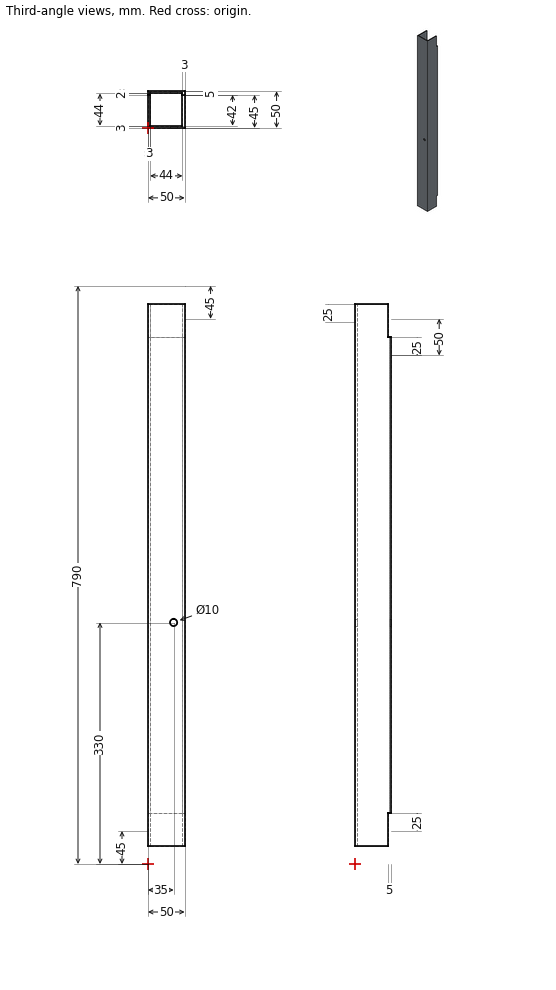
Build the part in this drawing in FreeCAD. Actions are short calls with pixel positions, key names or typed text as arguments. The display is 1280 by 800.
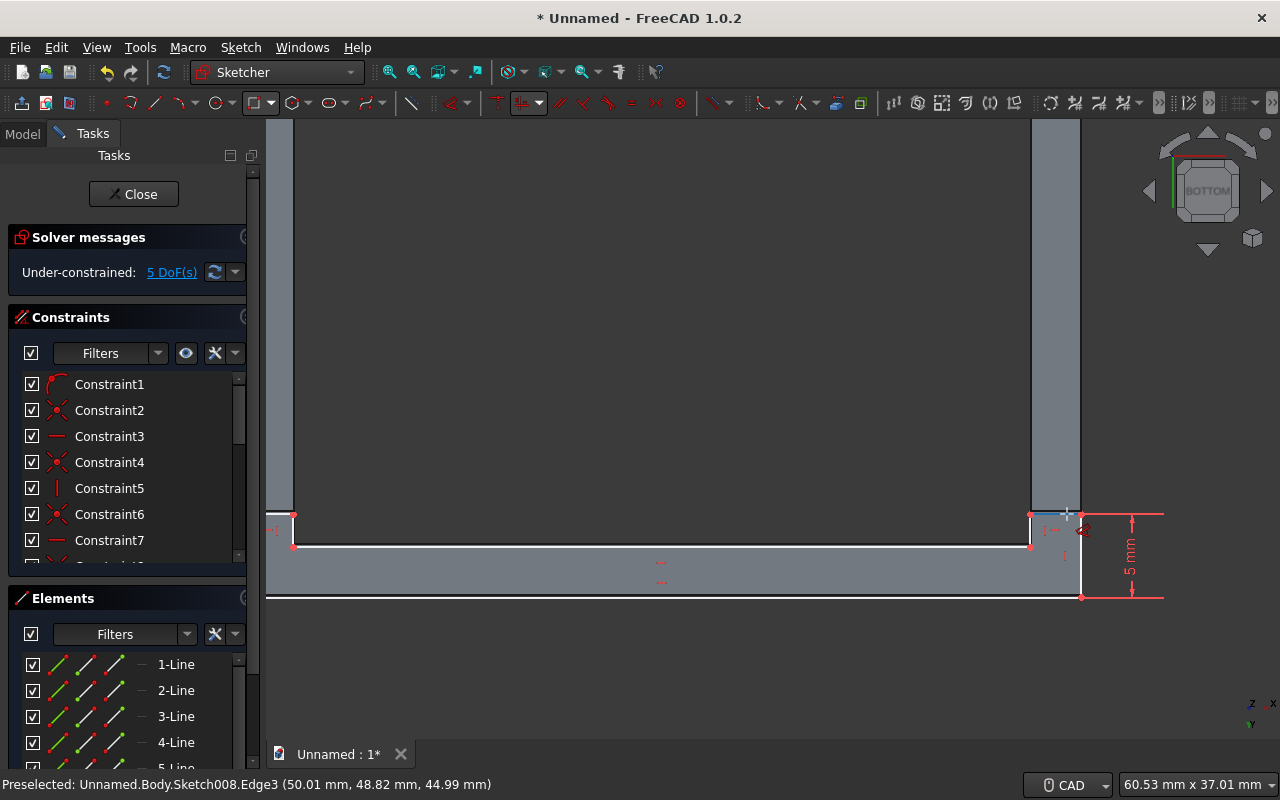
click(1066, 514)
click(1056, 548)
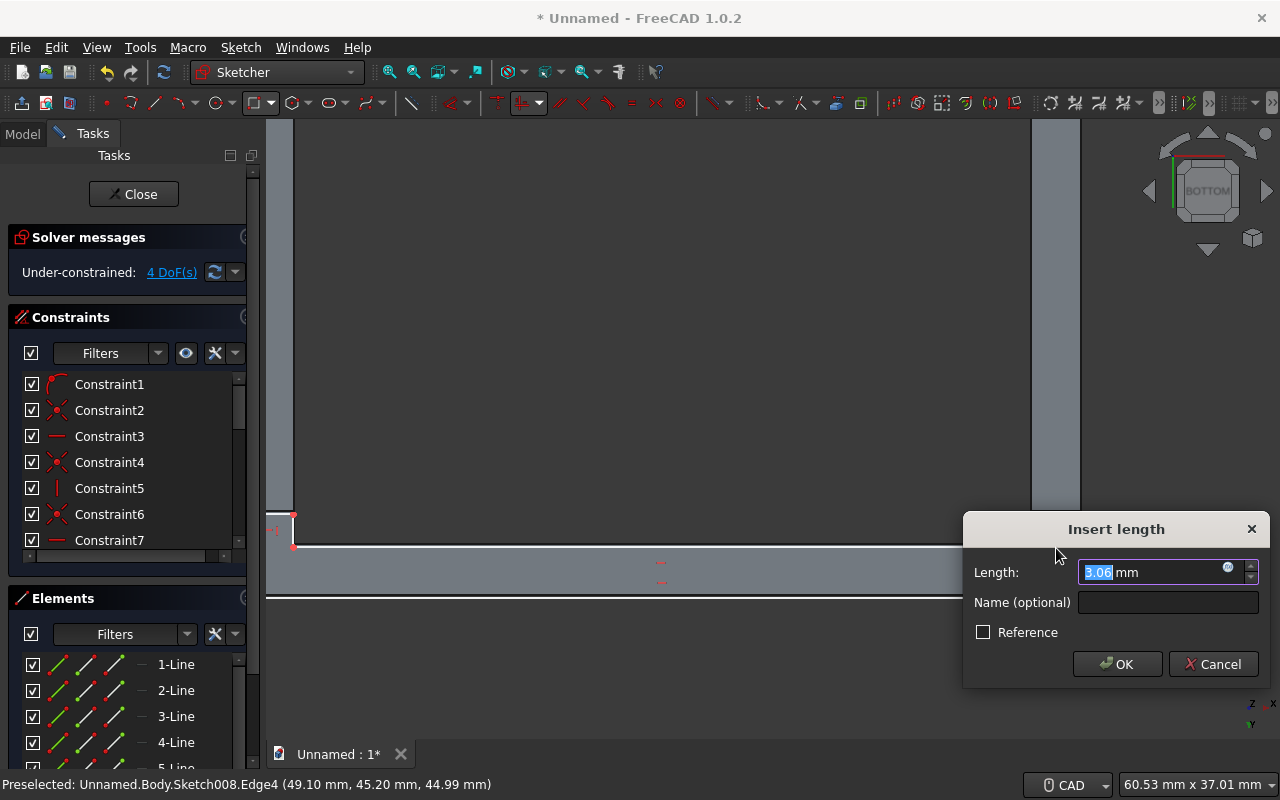
text(3)
key(Return)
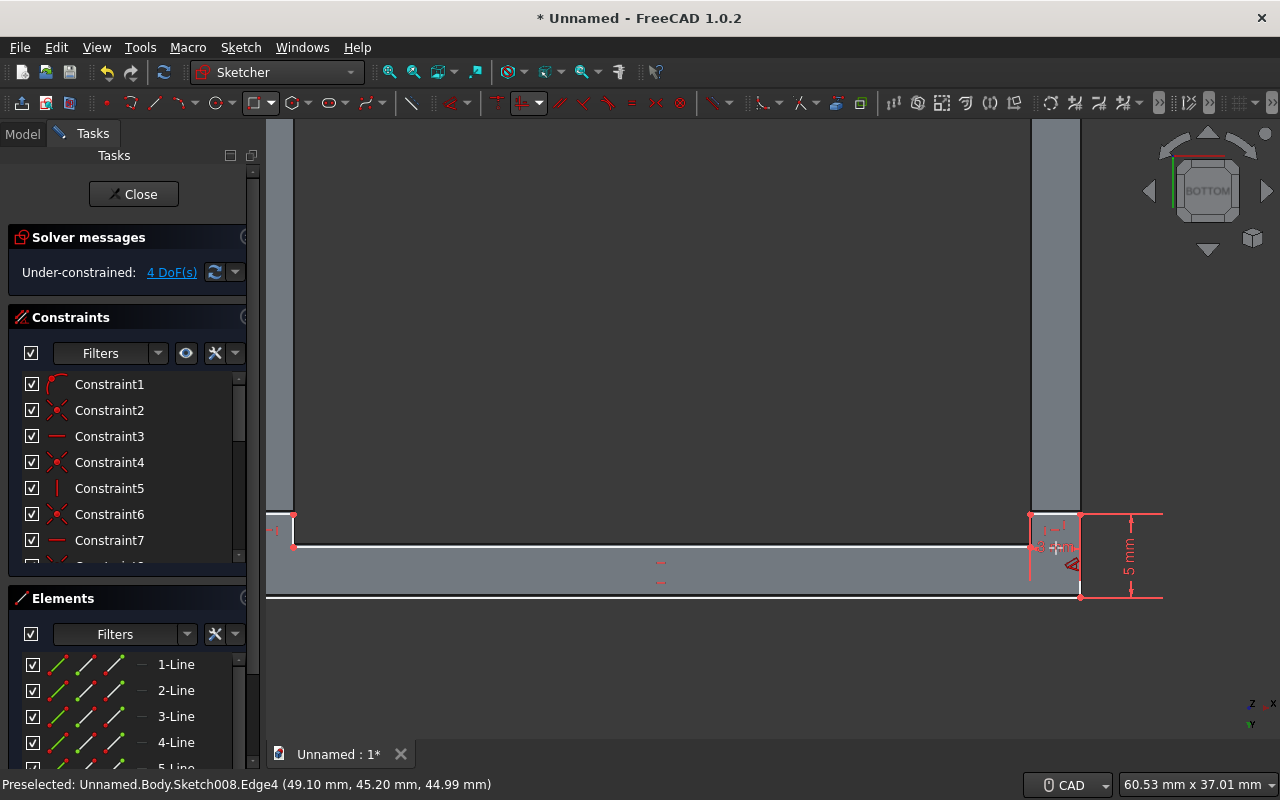
scroll(1030, 524, up, 2)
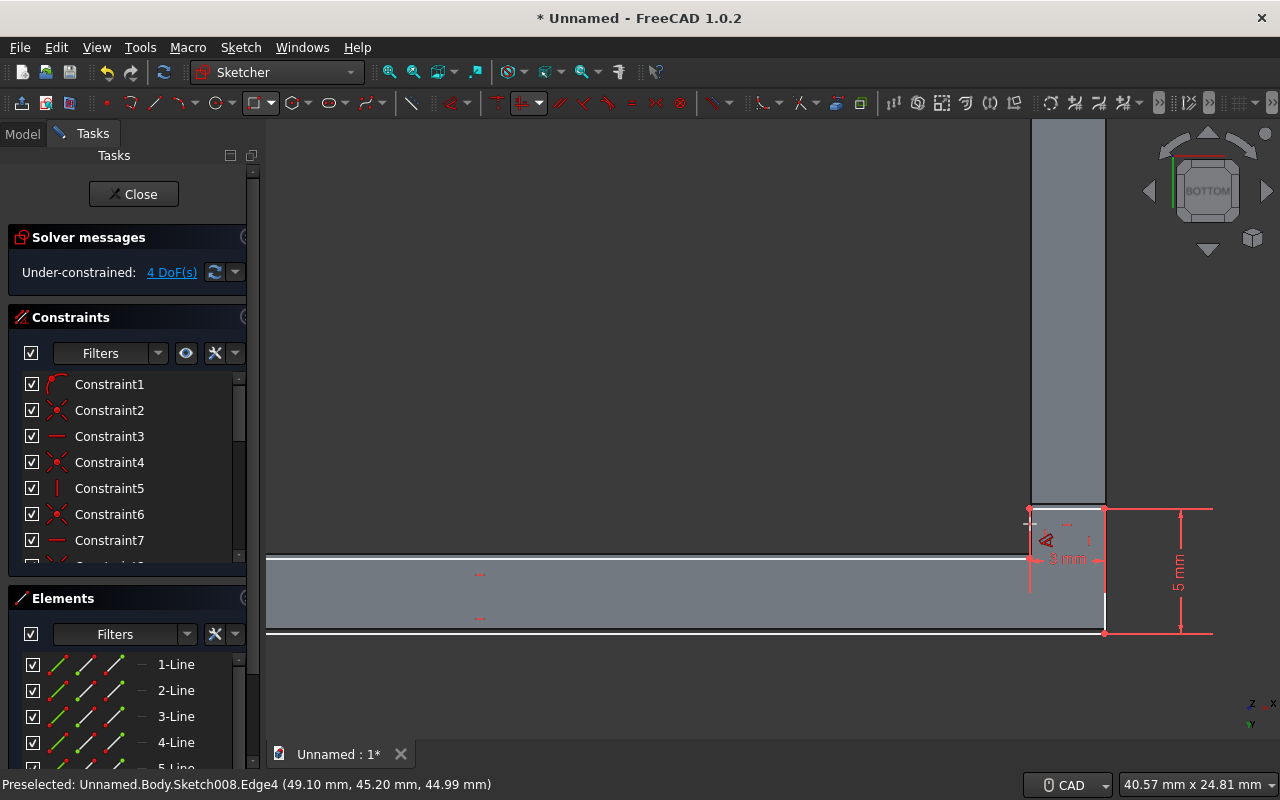
click(1030, 524)
click(1064, 534)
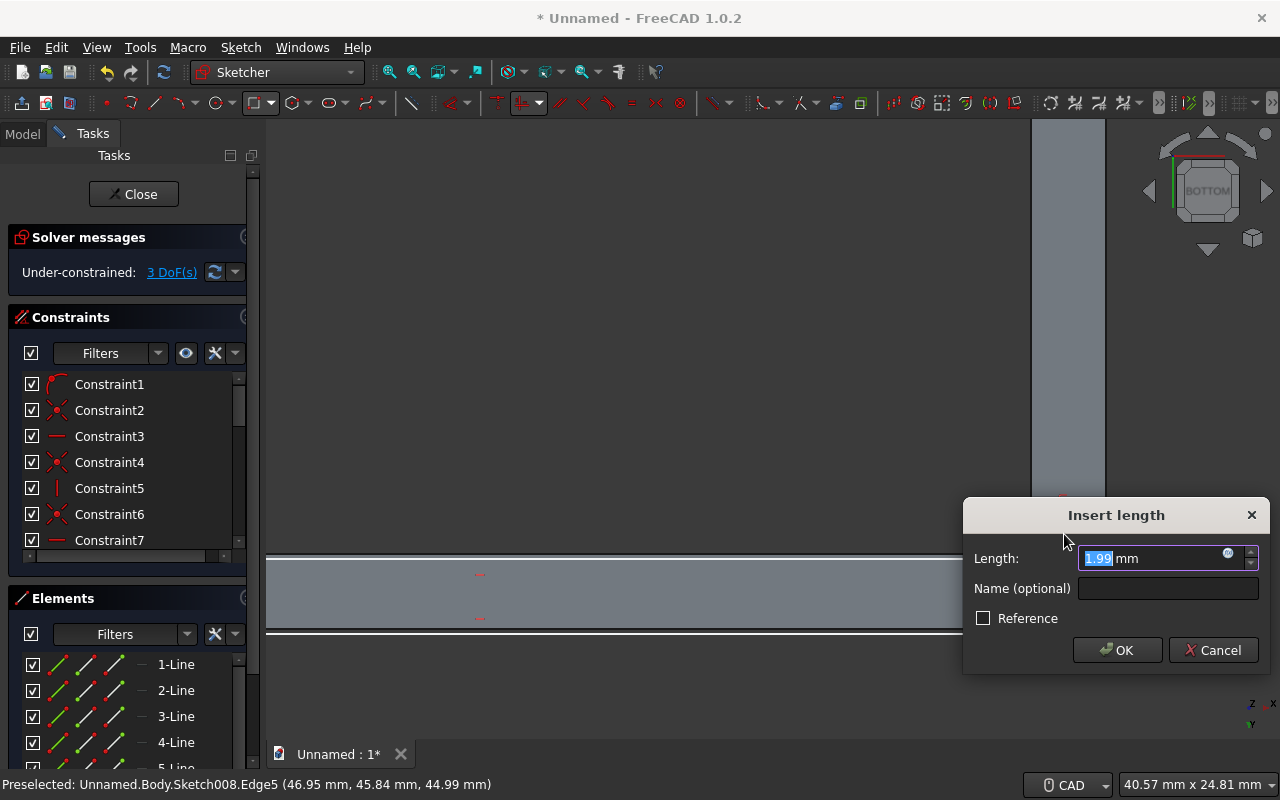
text(2)
key(Return)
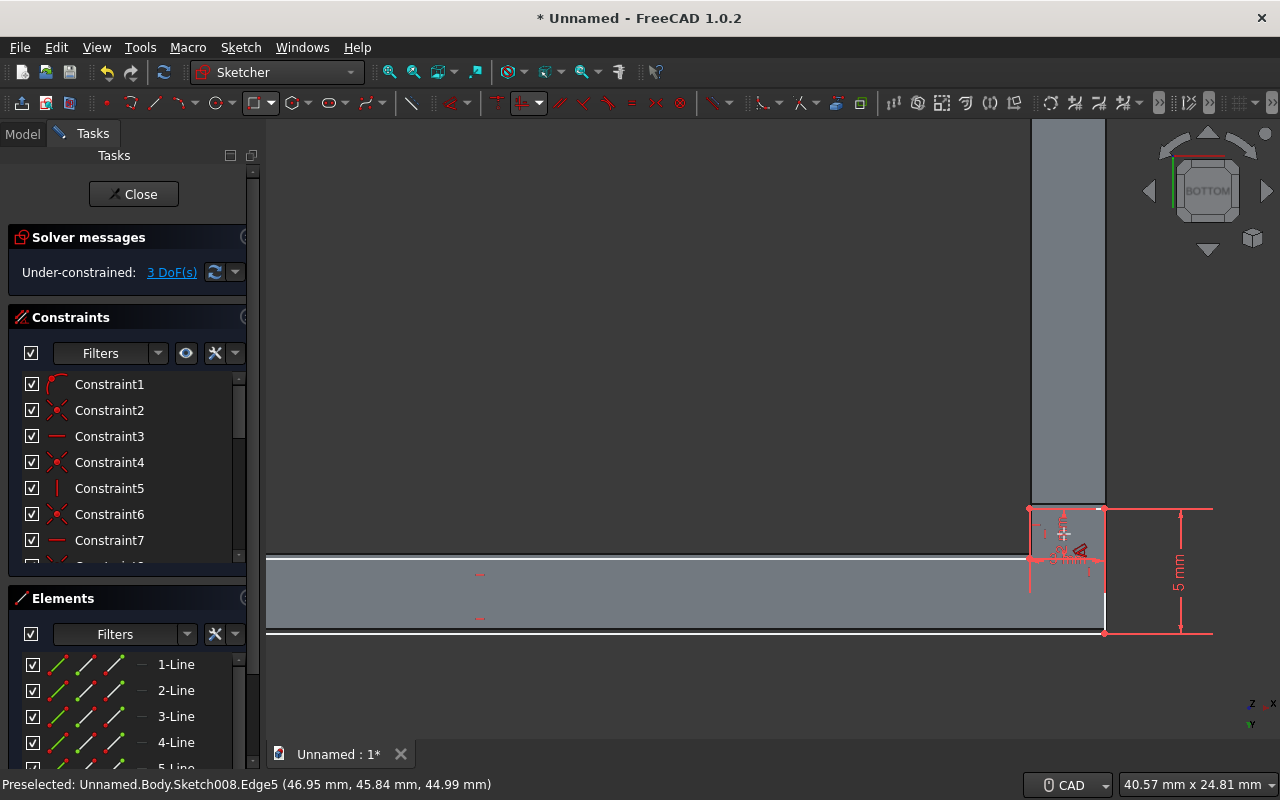
scroll(801, 612, down, 6)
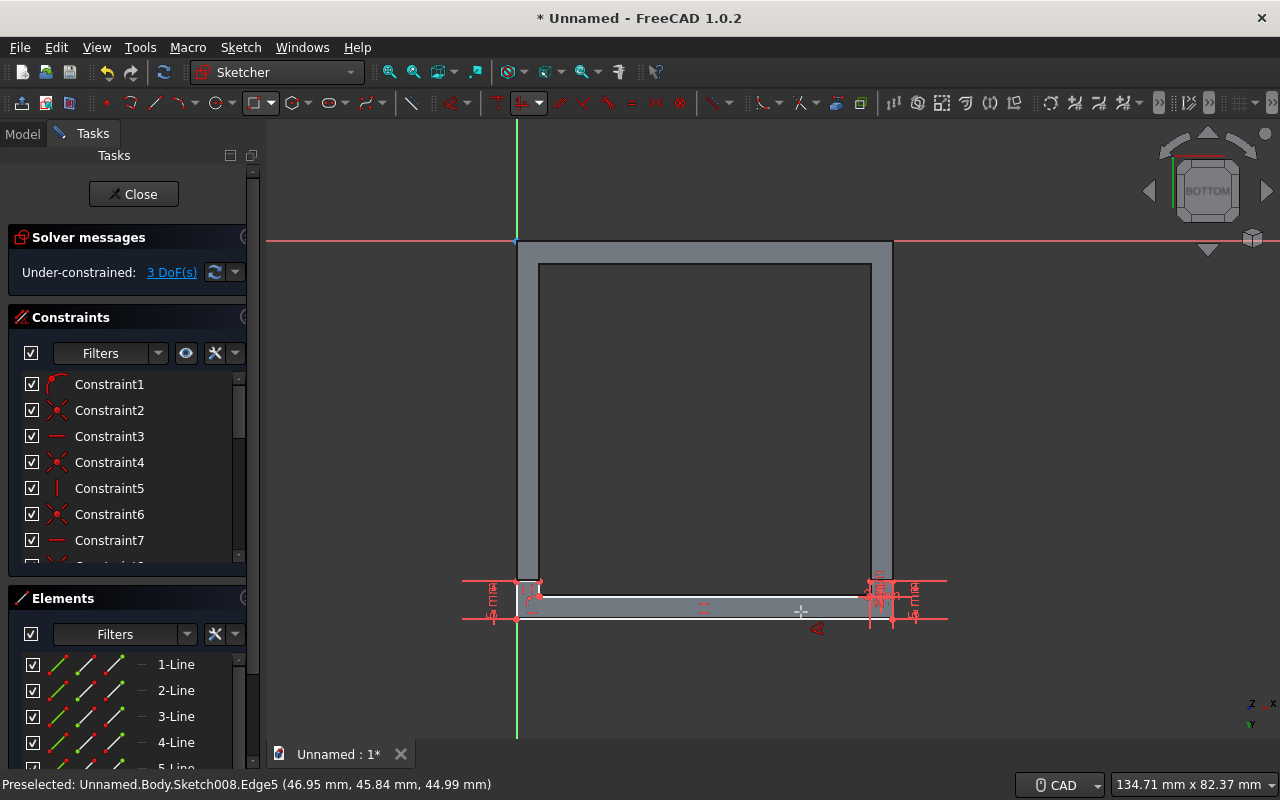
scroll(533, 581, up, 4)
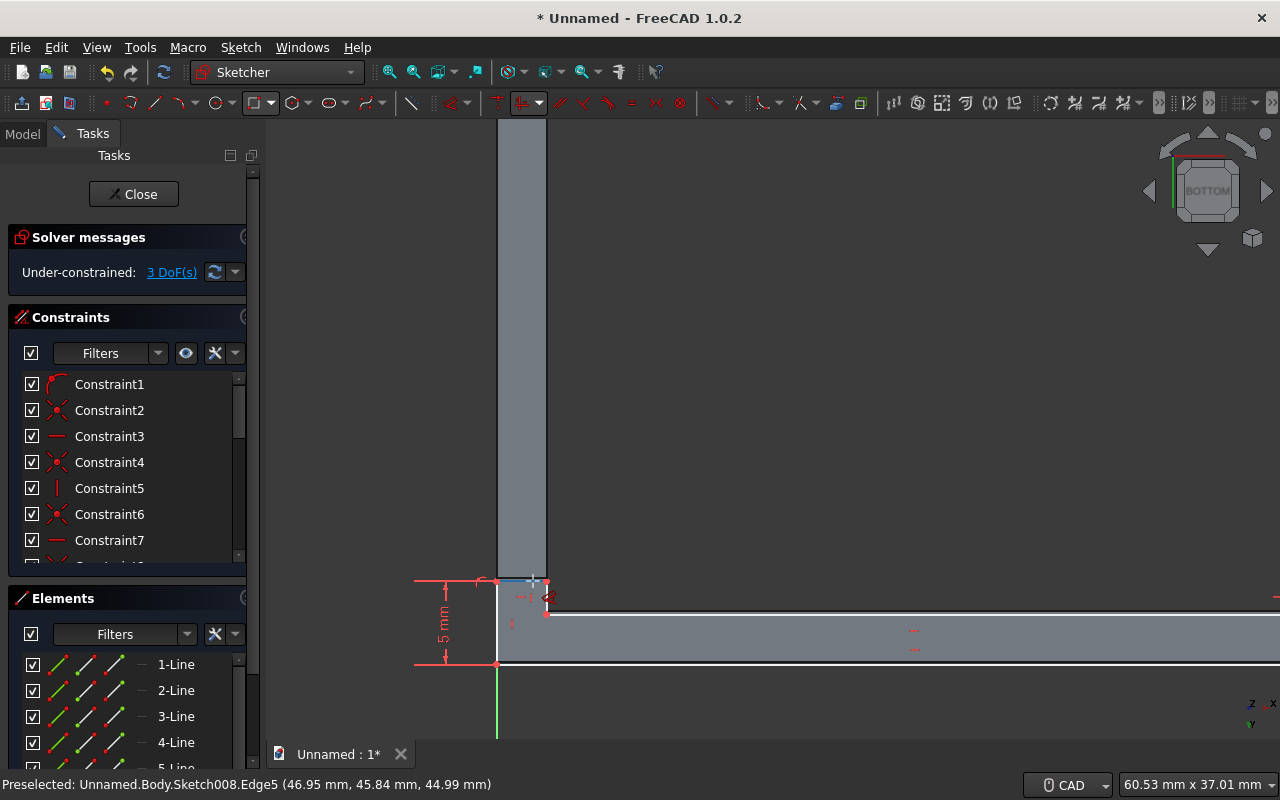
click(532, 581)
click(522, 615)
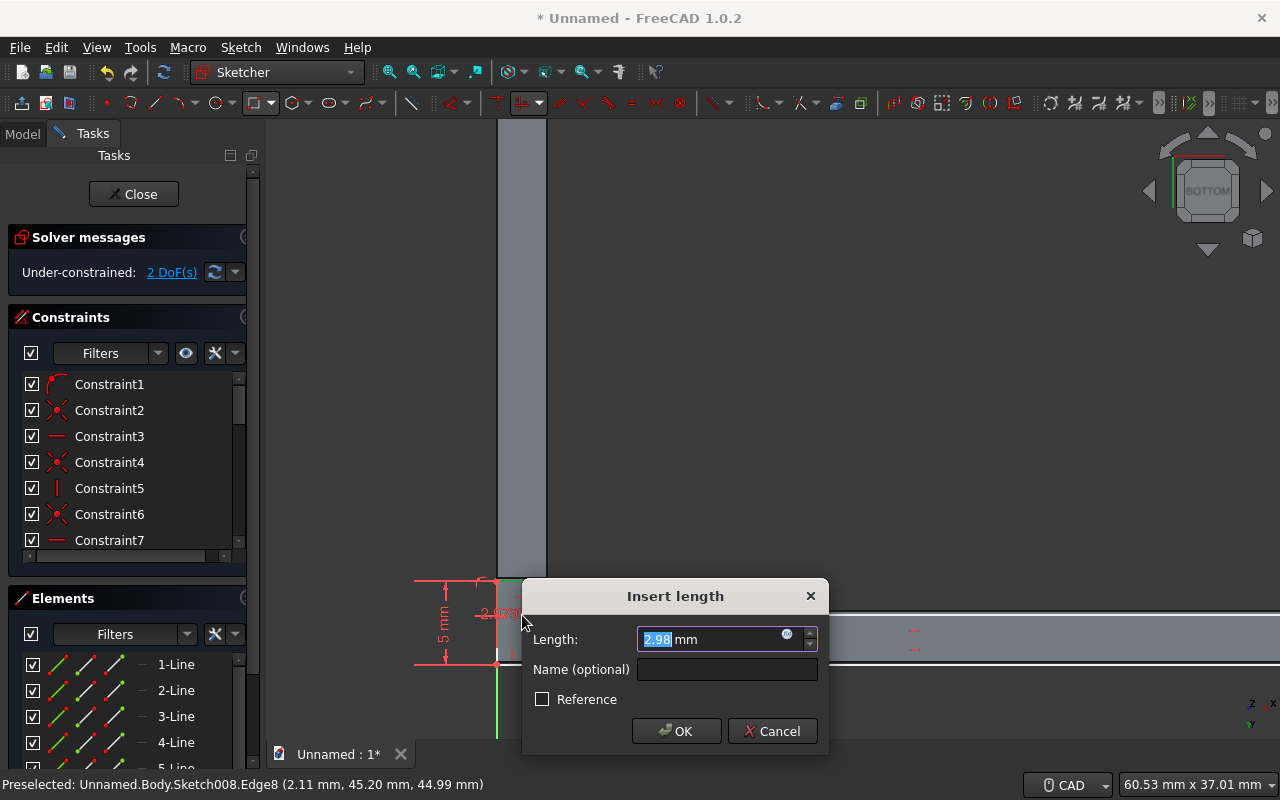
text(3)
key(Return)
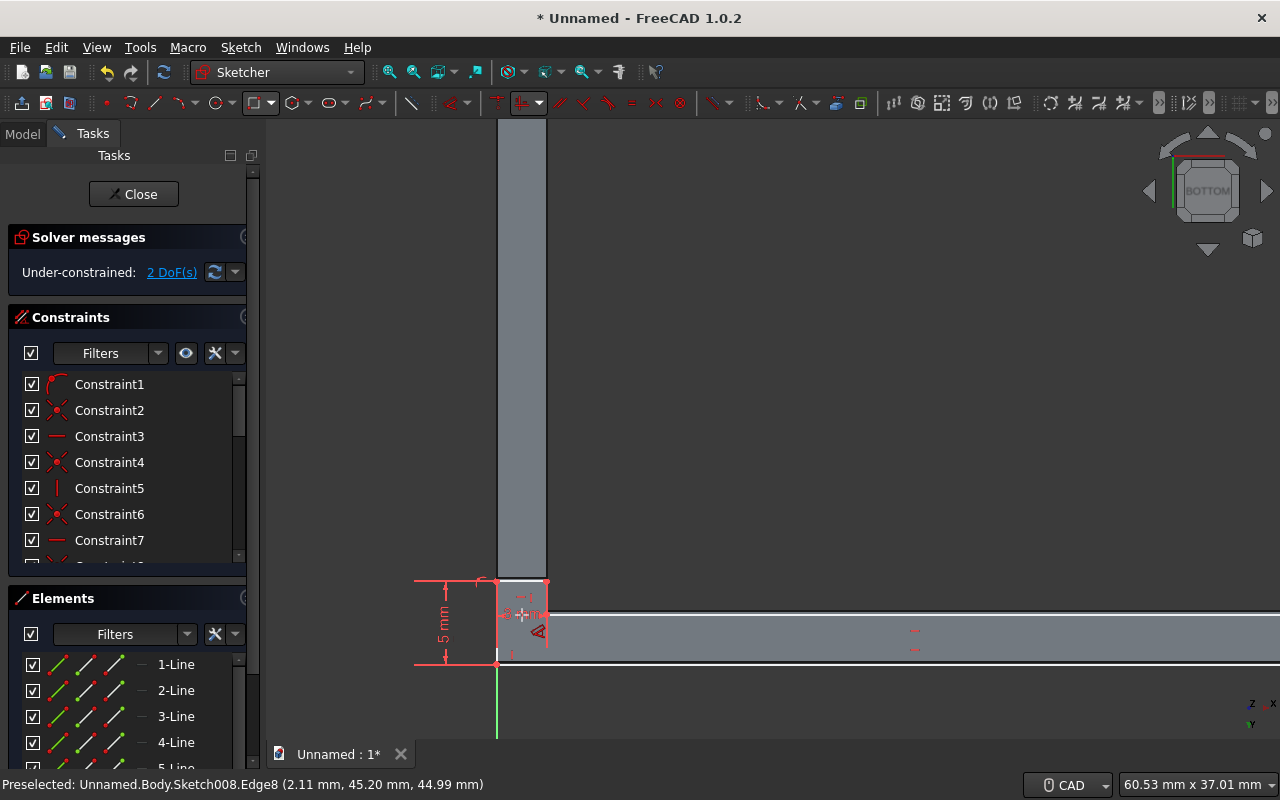
click(748, 665)
click(806, 699)